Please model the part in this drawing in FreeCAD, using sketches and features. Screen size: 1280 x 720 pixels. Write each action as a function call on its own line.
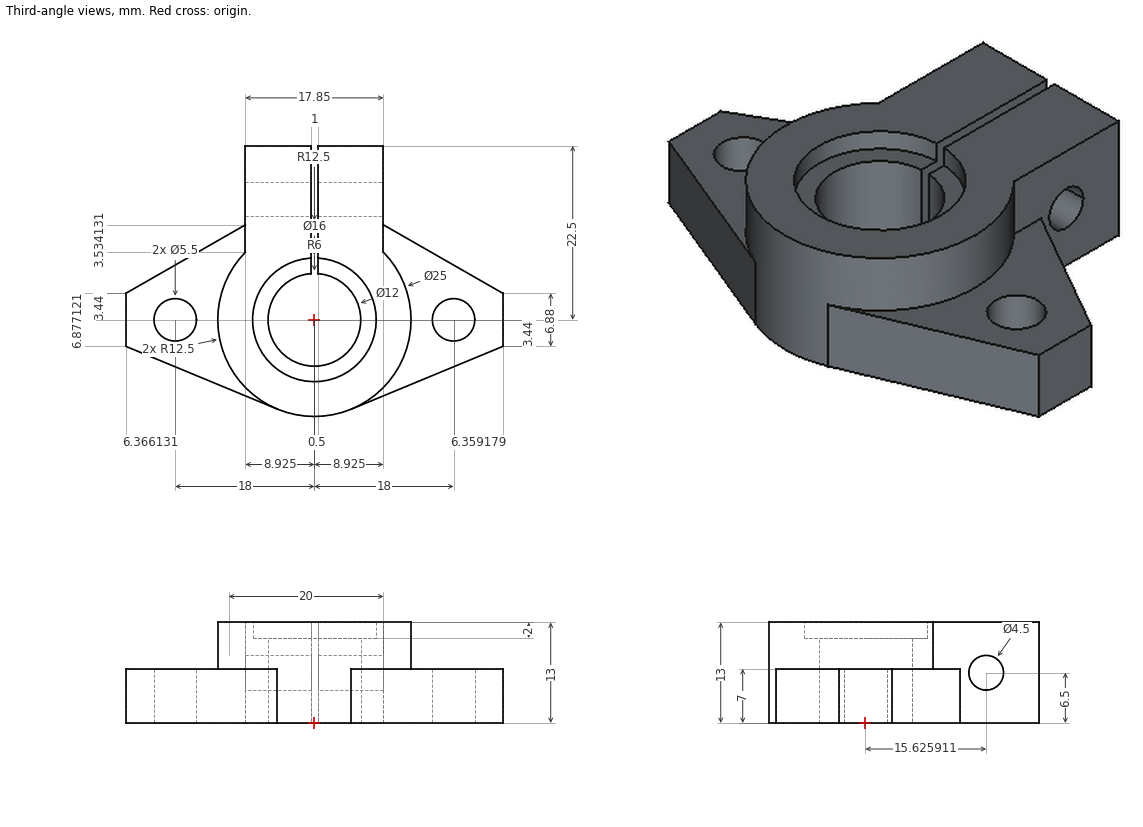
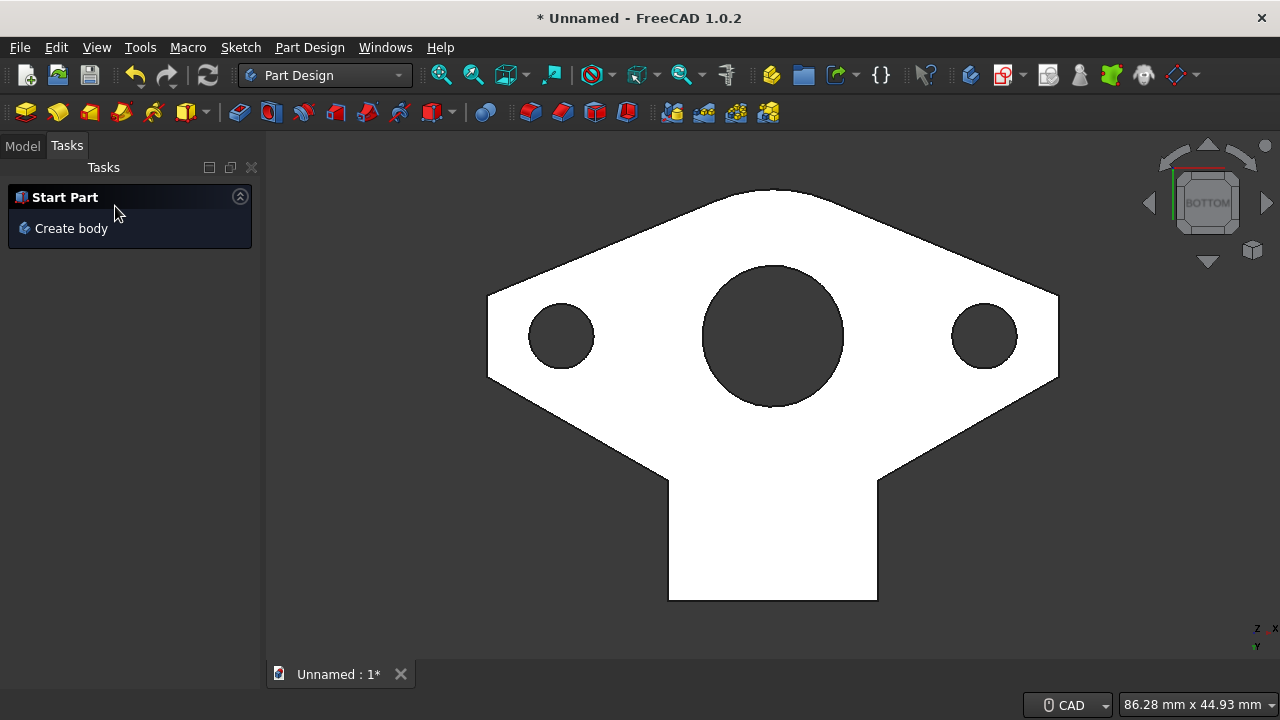
key(0)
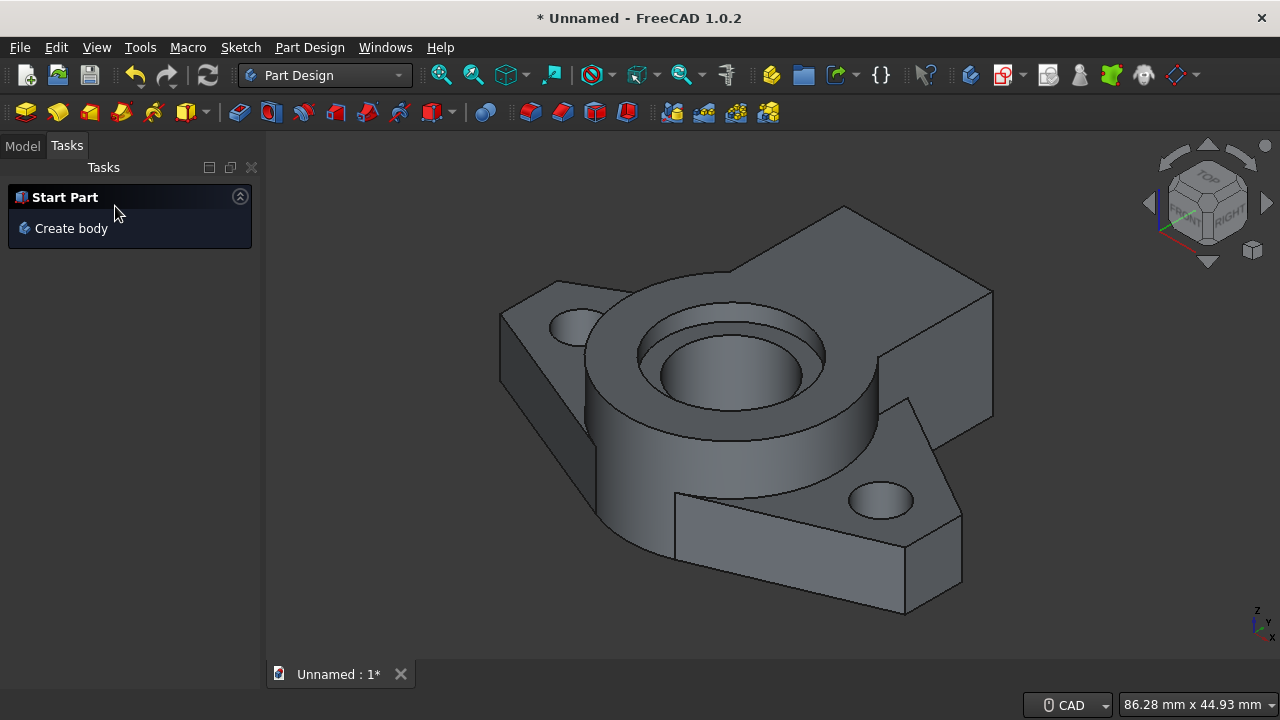
click(856, 284)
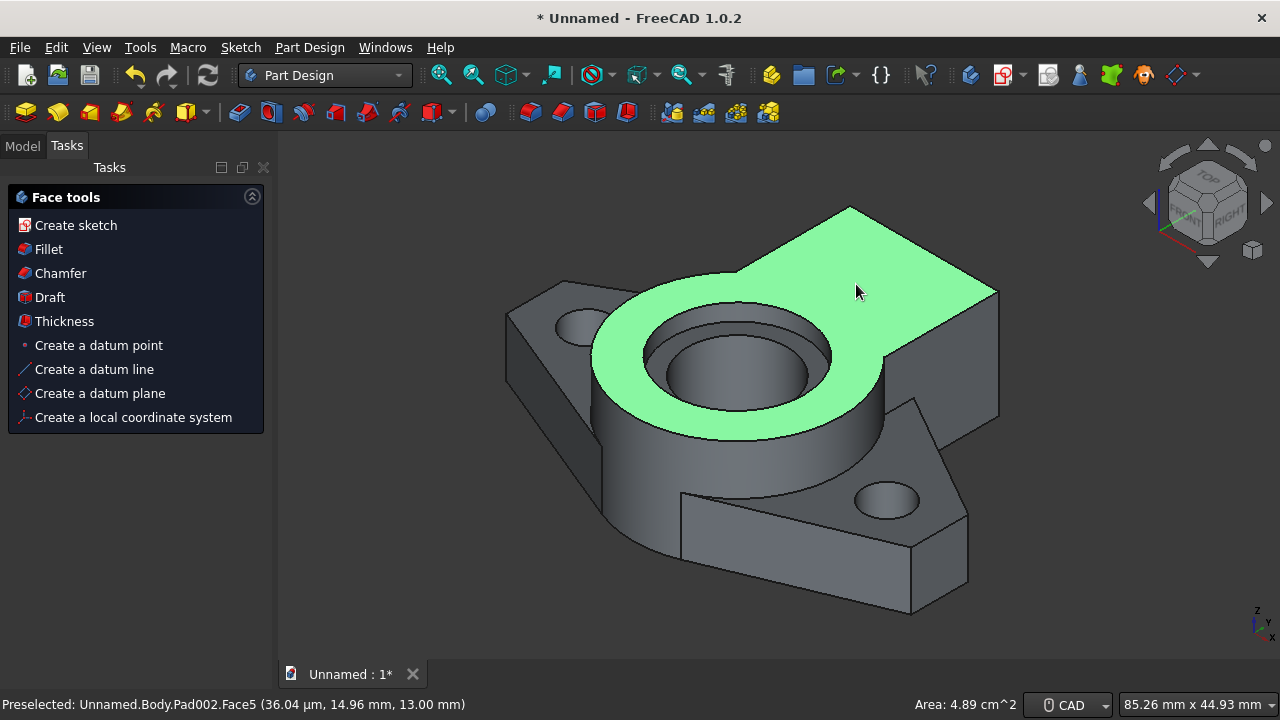
click(1004, 76)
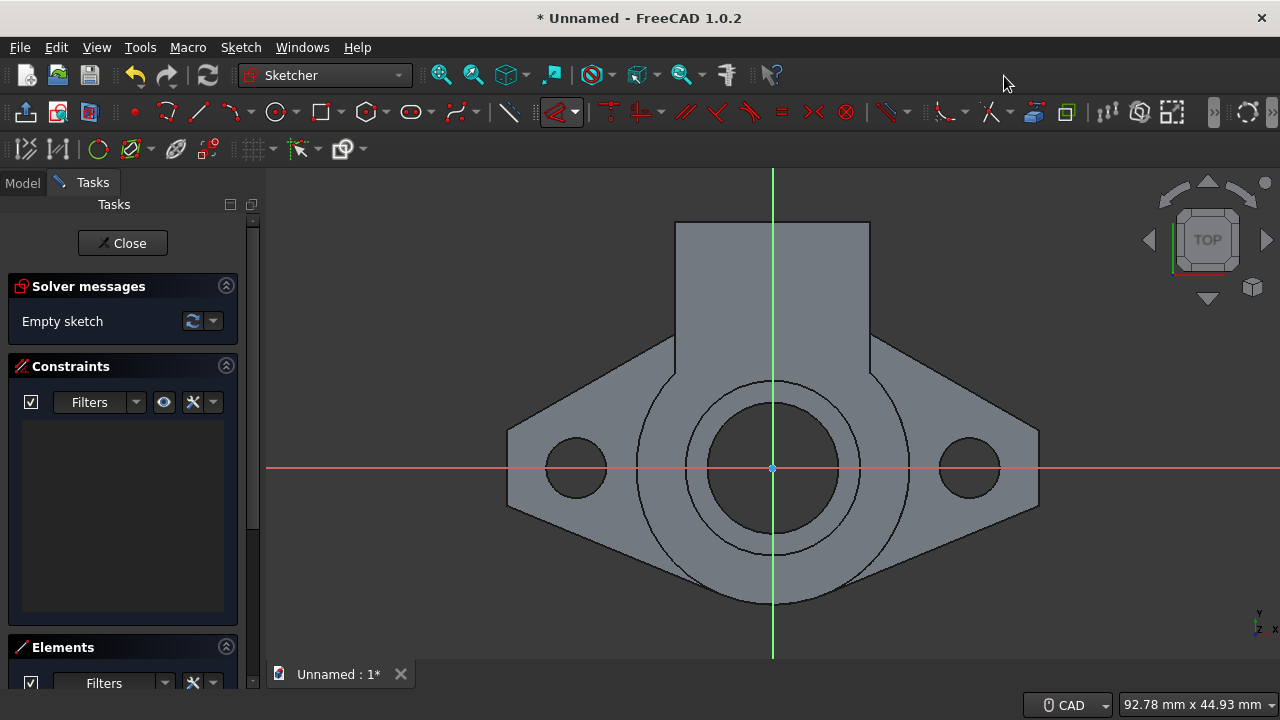
click(168, 112)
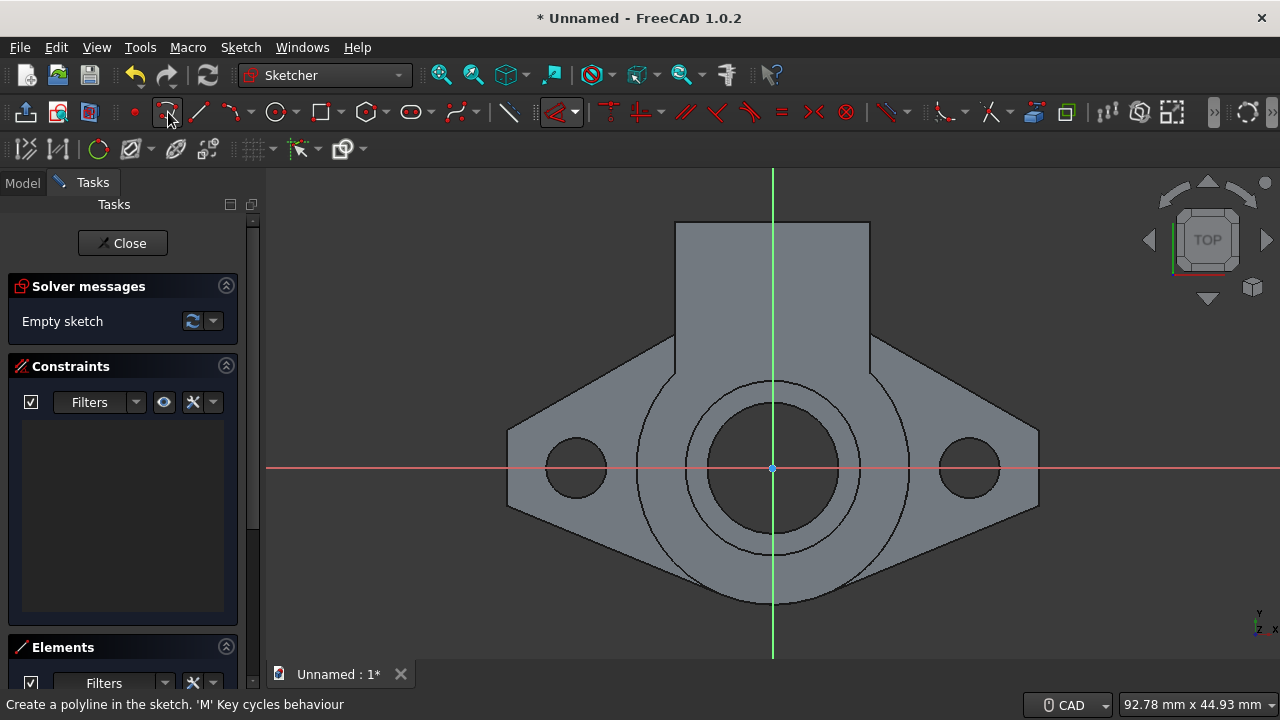
scroll(778, 403, up, 6)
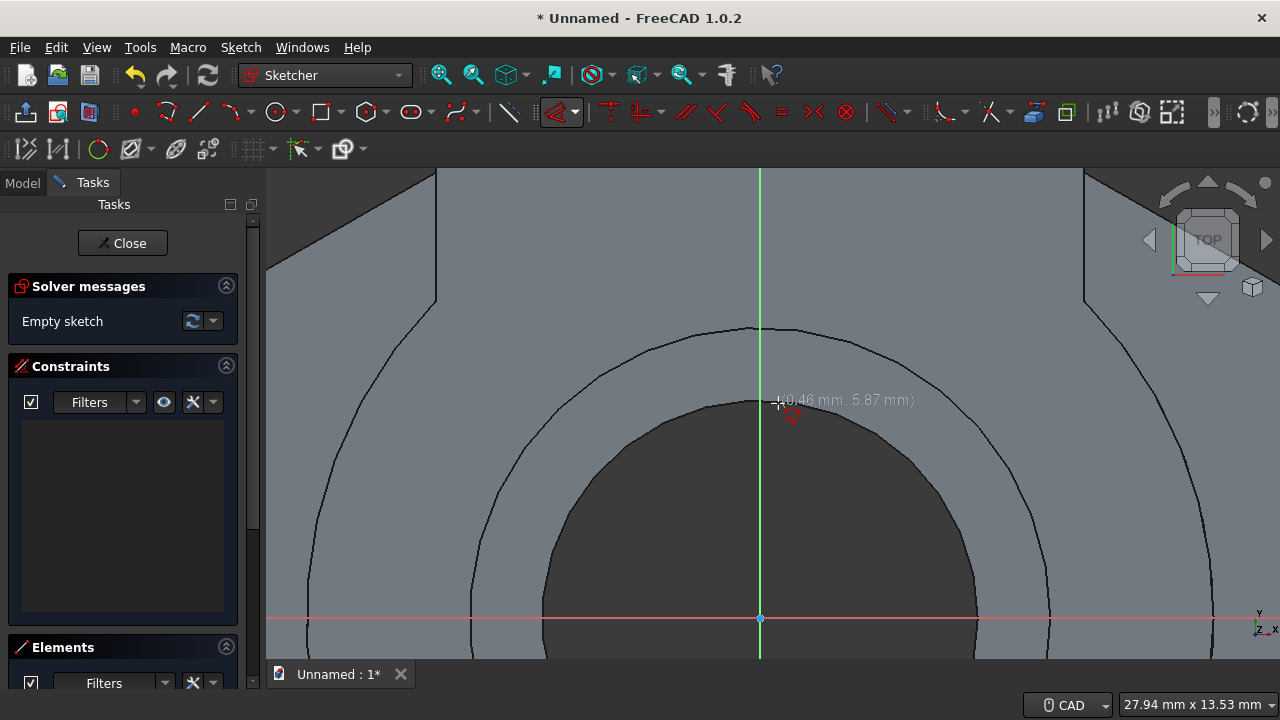
click(778, 401)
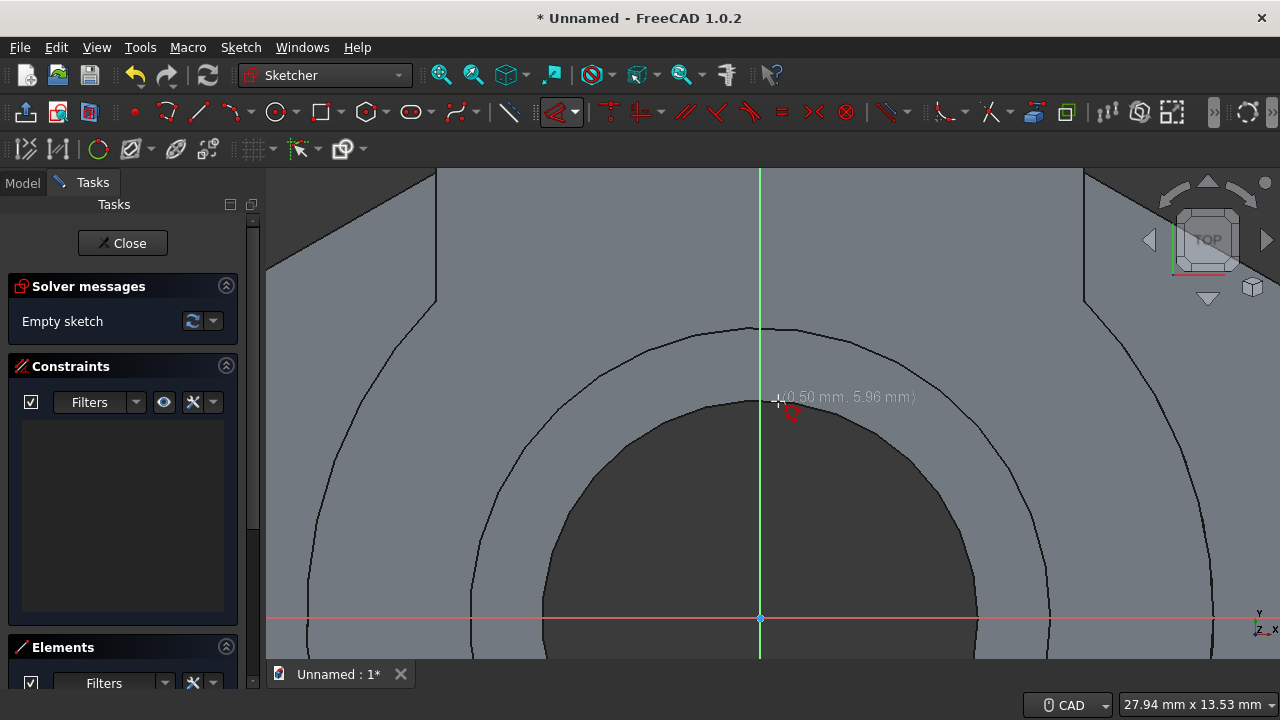
scroll(672, 532, down, 5)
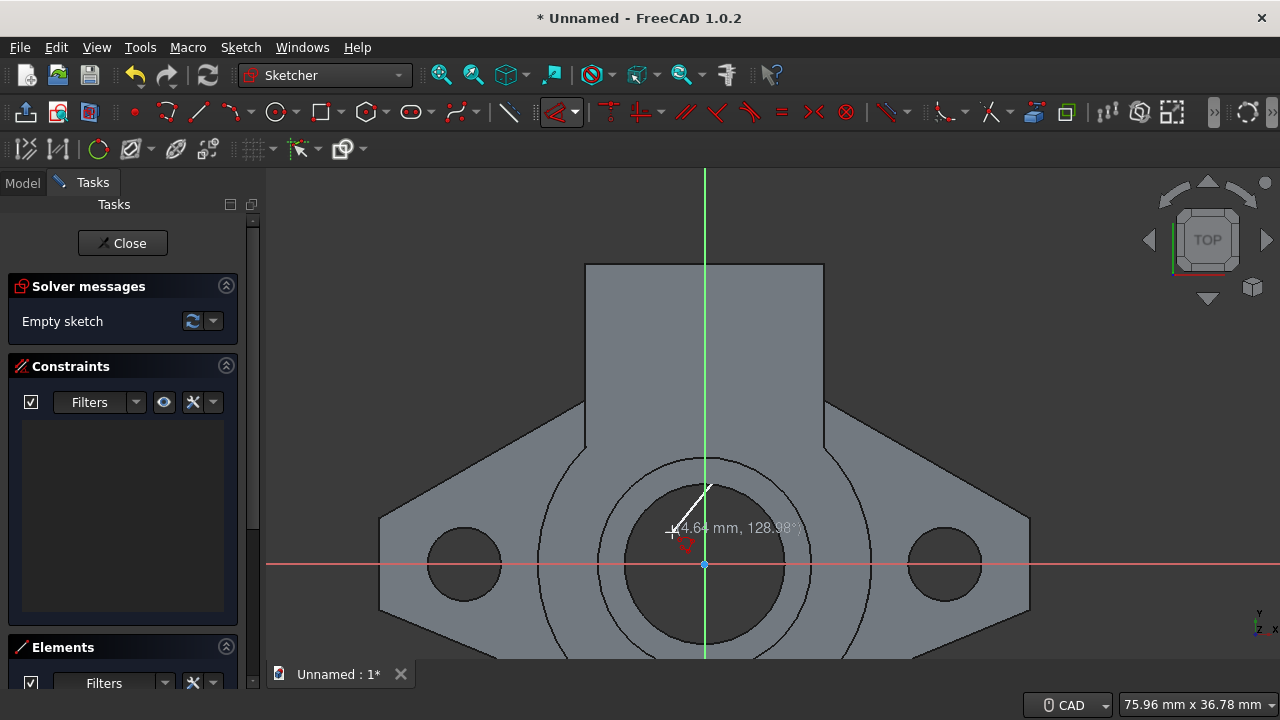
scroll(711, 264, up, 5)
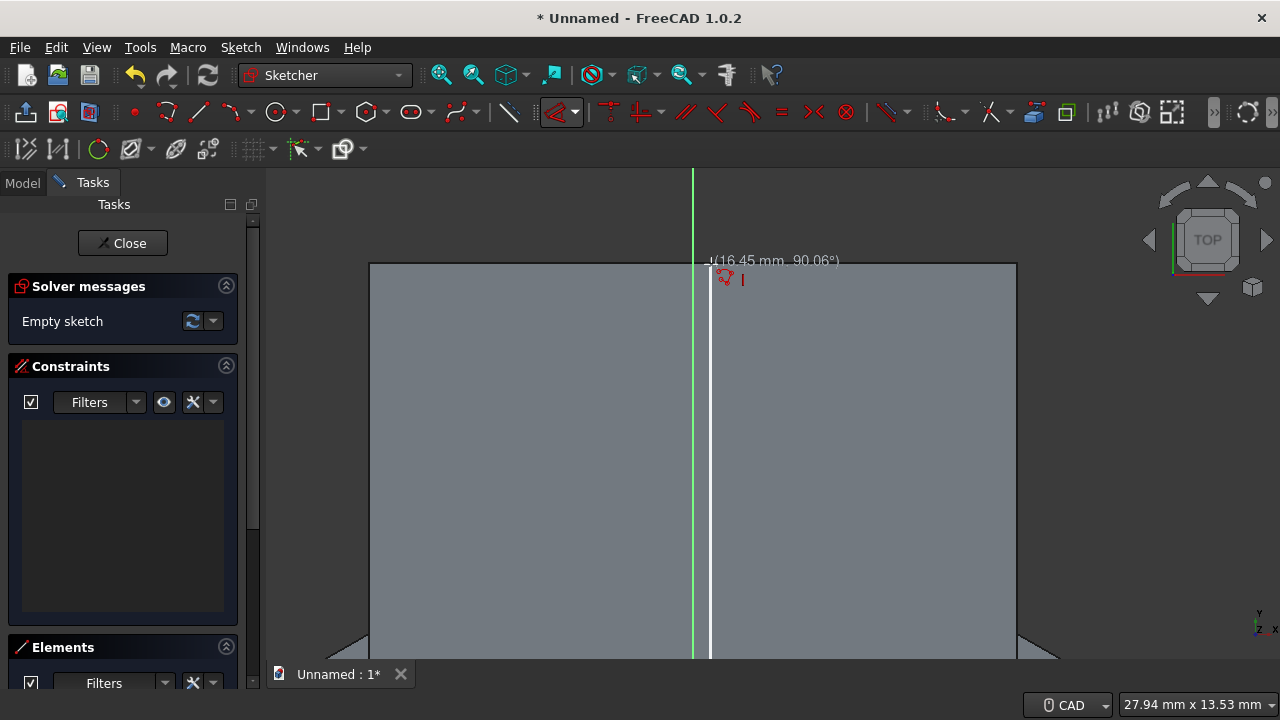
click(711, 263)
click(675, 263)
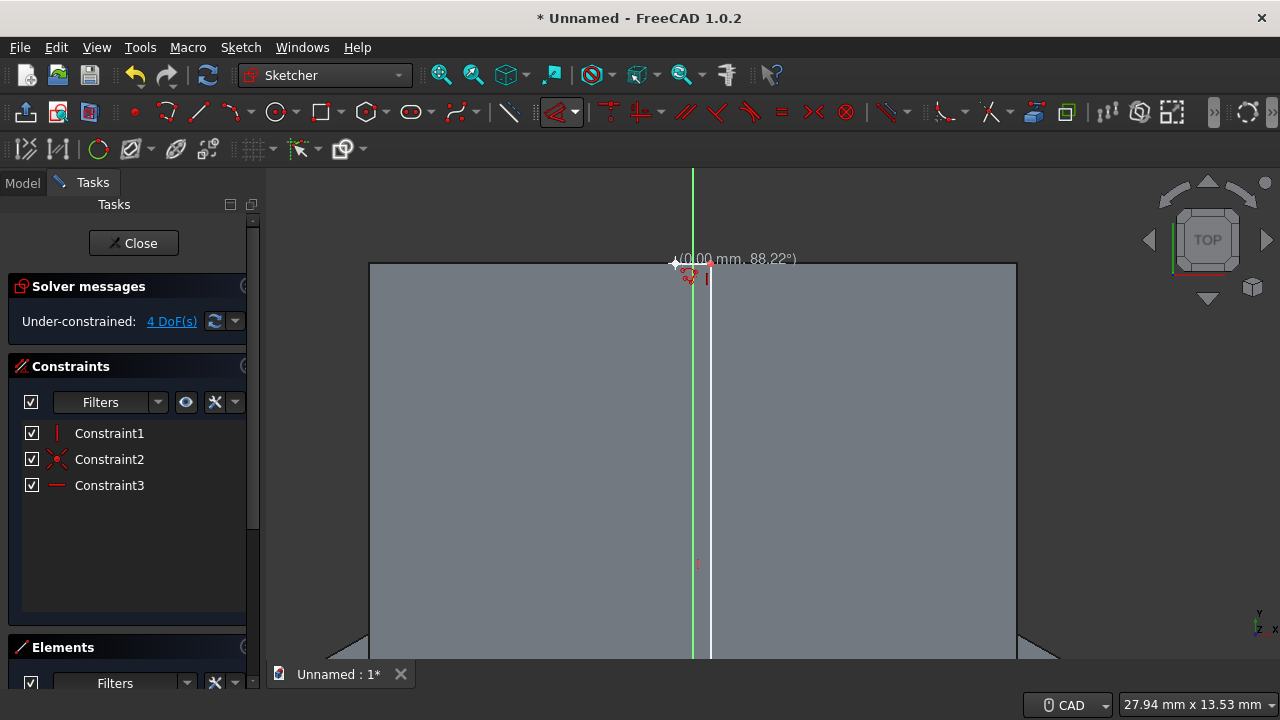
scroll(711, 263, down, 5)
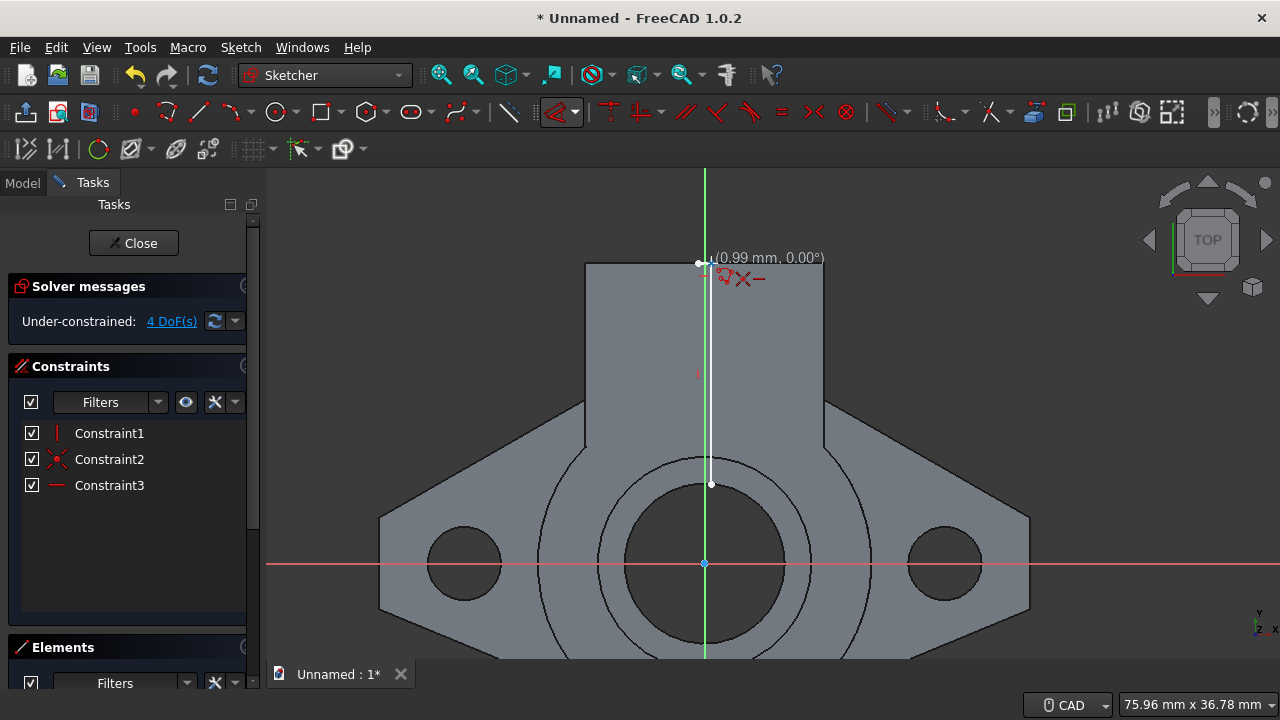
scroll(698, 484, up, 5)